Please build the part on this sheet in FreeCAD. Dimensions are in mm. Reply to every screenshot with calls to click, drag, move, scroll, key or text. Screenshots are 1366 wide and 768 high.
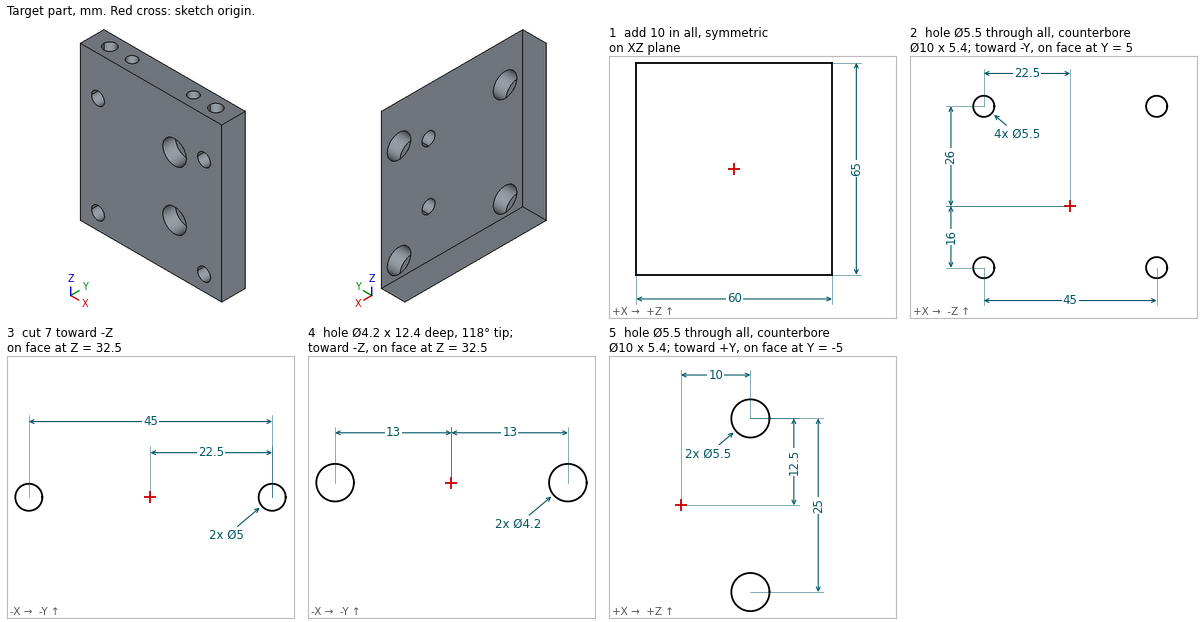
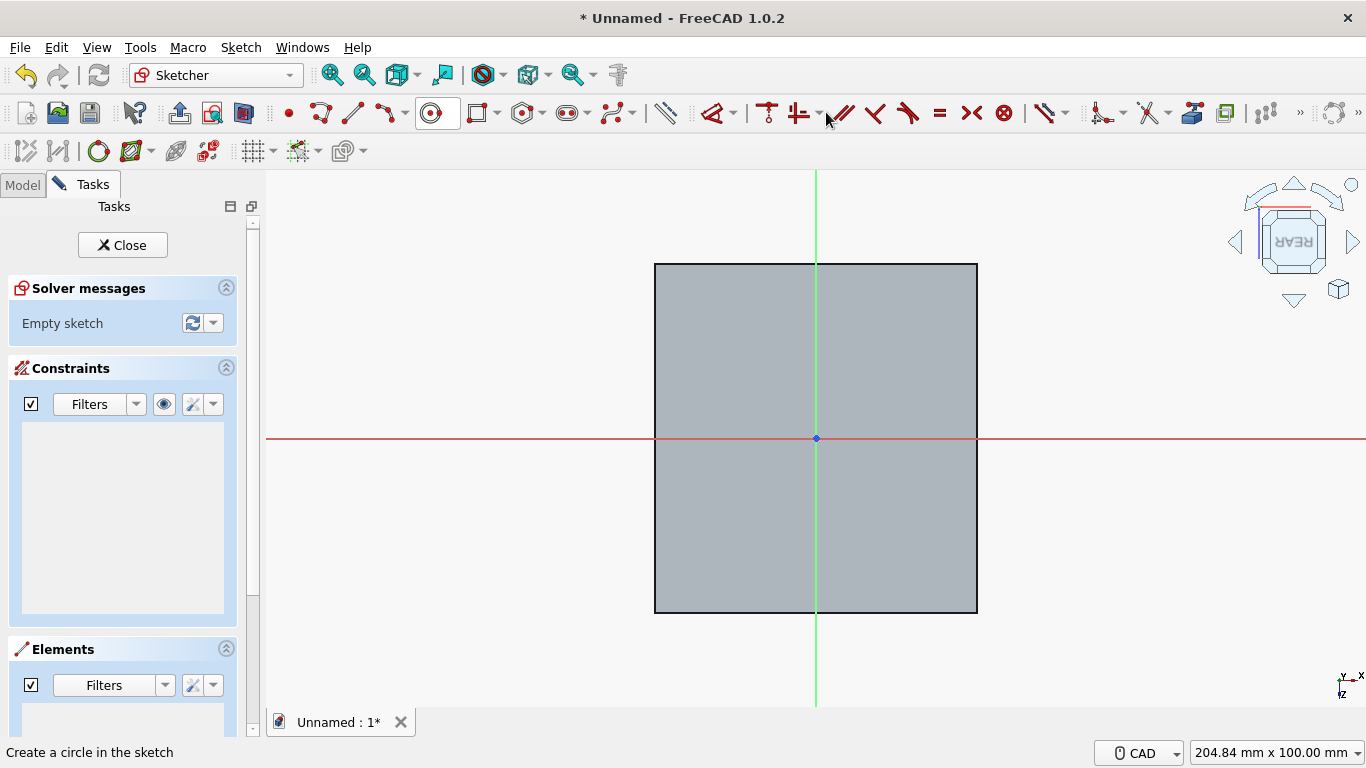
key(g)
key(c)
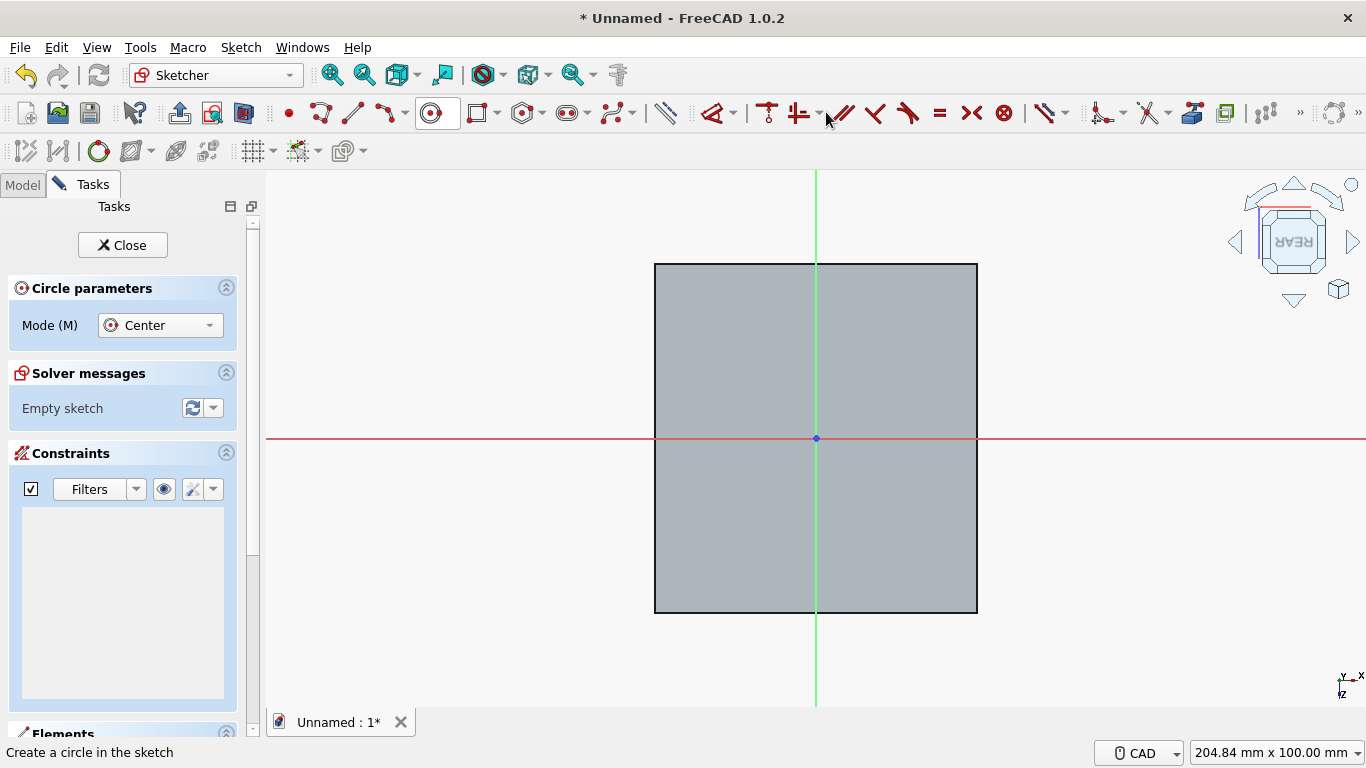
scroll(695, 299, up, 3)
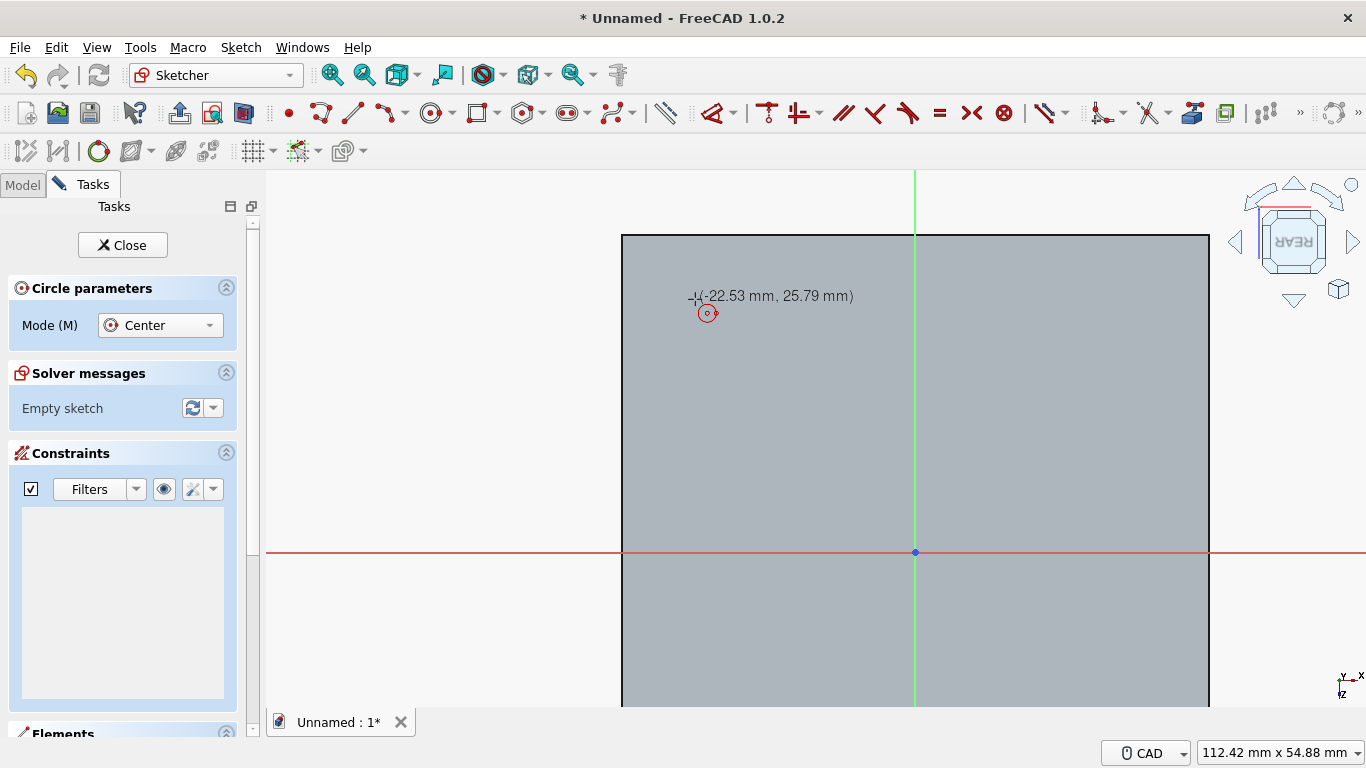
click(695, 299)
click(714, 280)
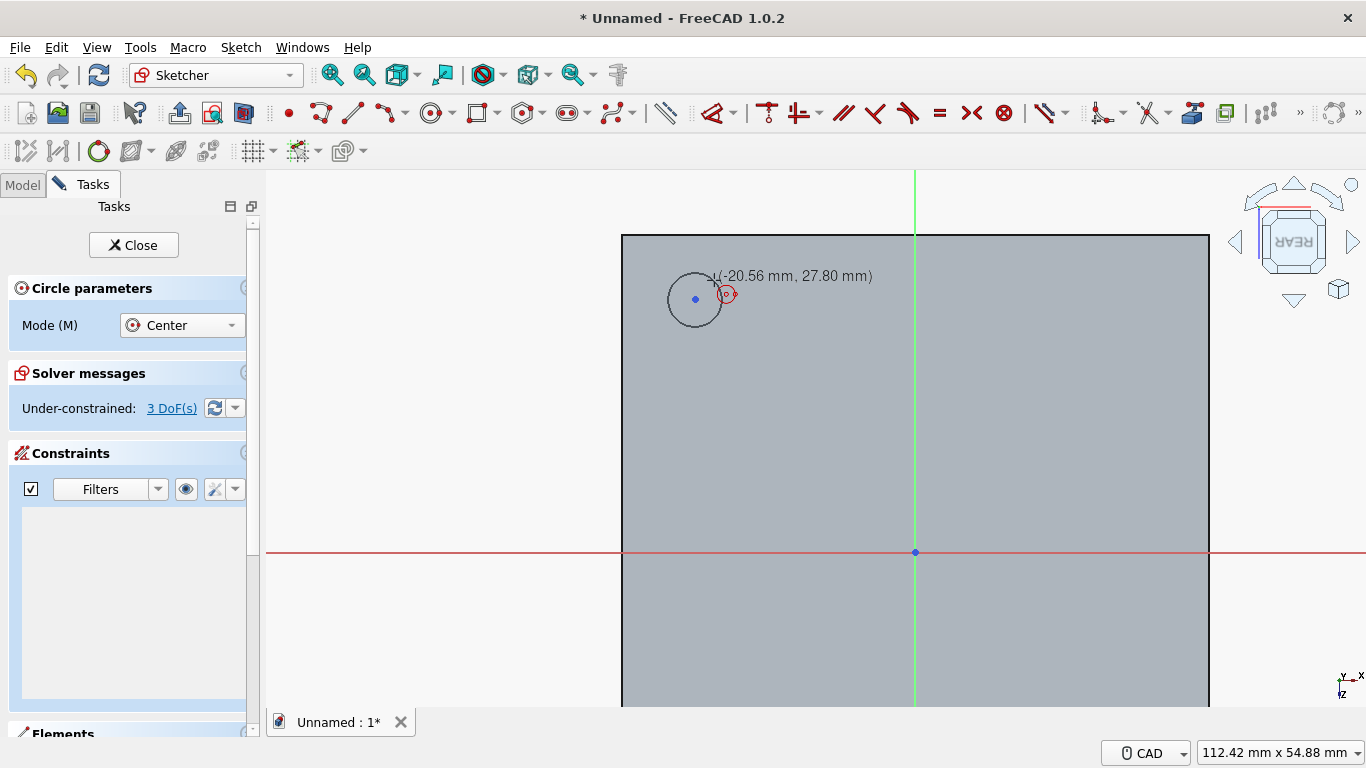
scroll(407, 305, down, 2)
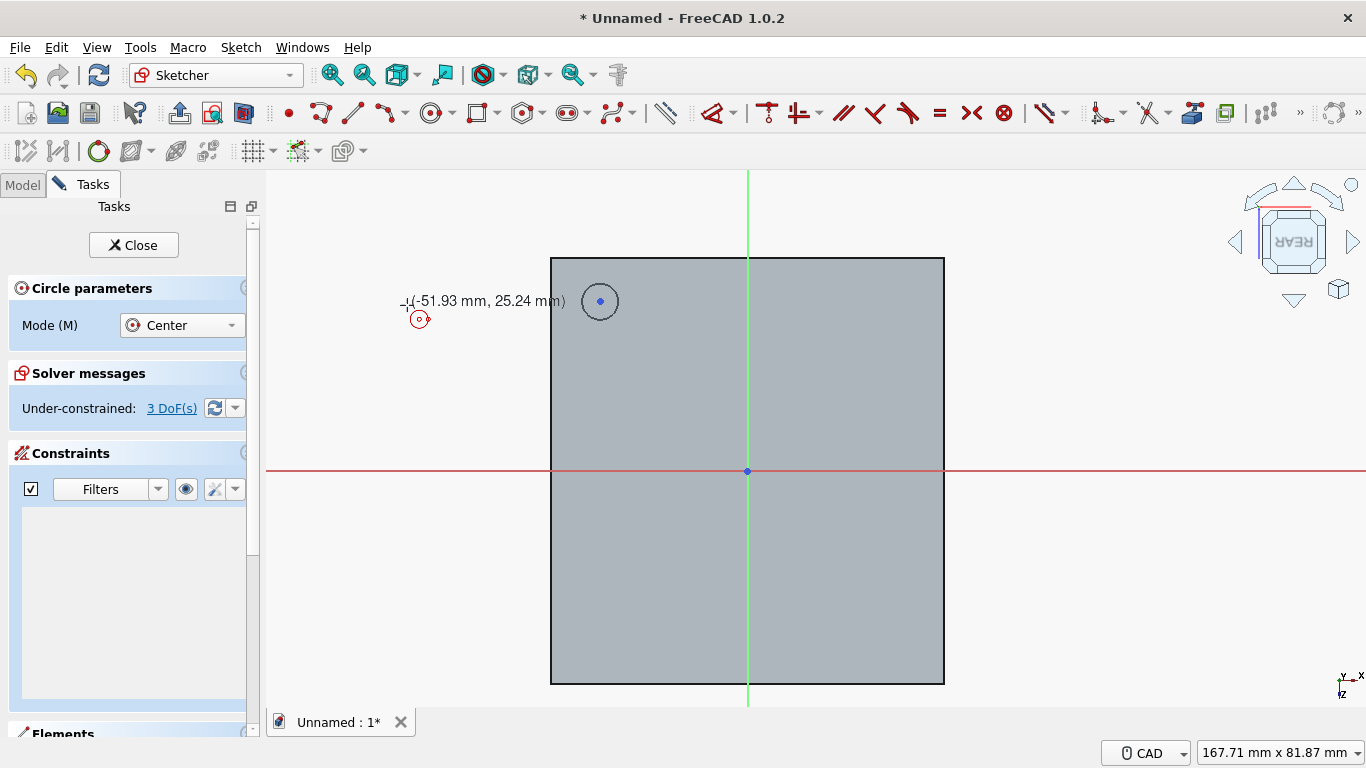
scroll(600, 576, up, 2)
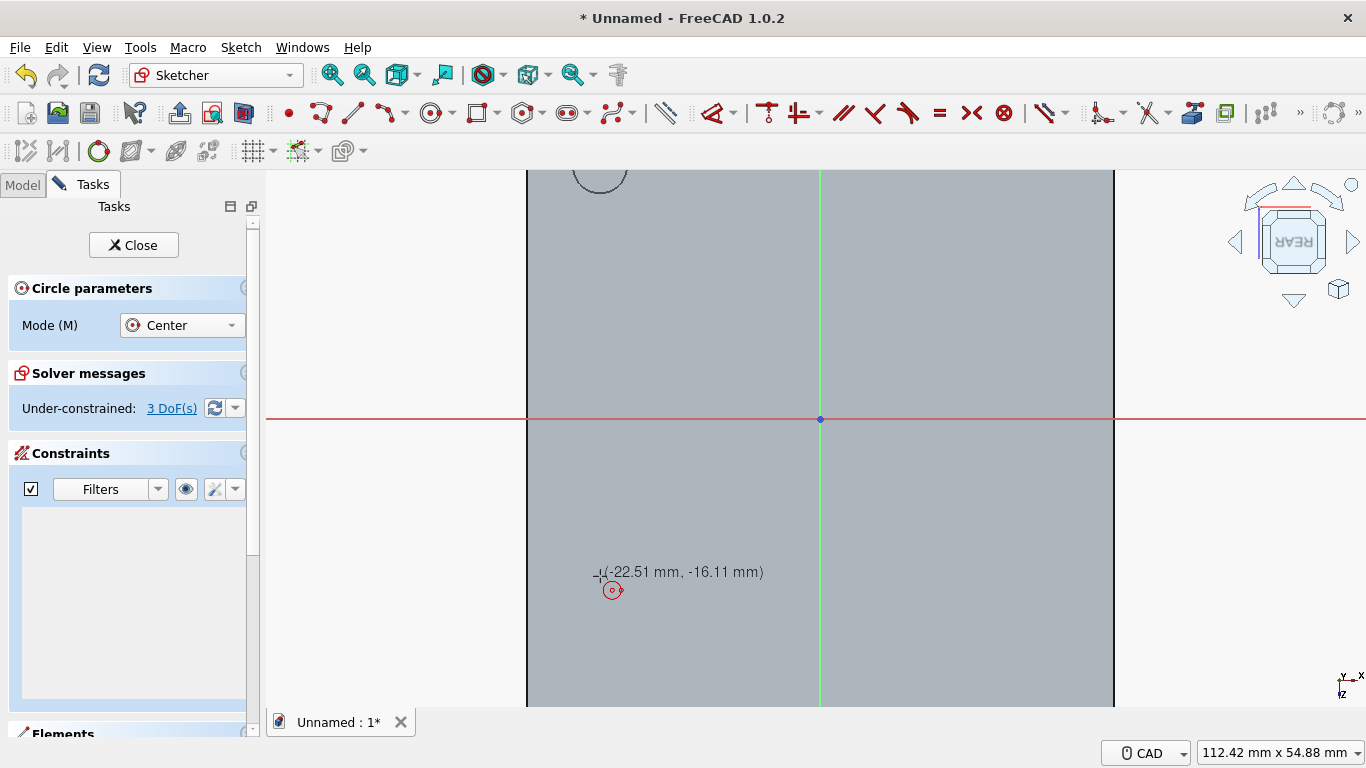
click(600, 576)
click(619, 557)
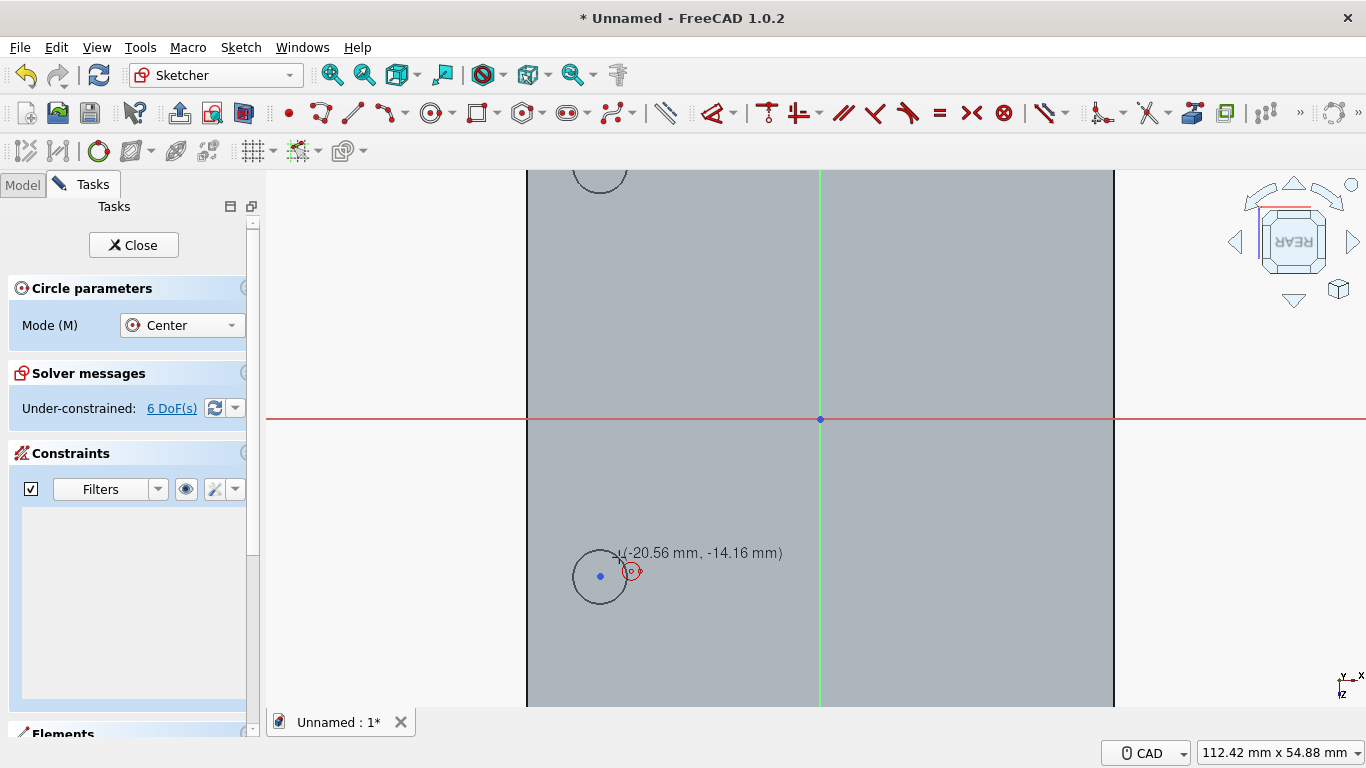
click(1040, 576)
click(1059, 557)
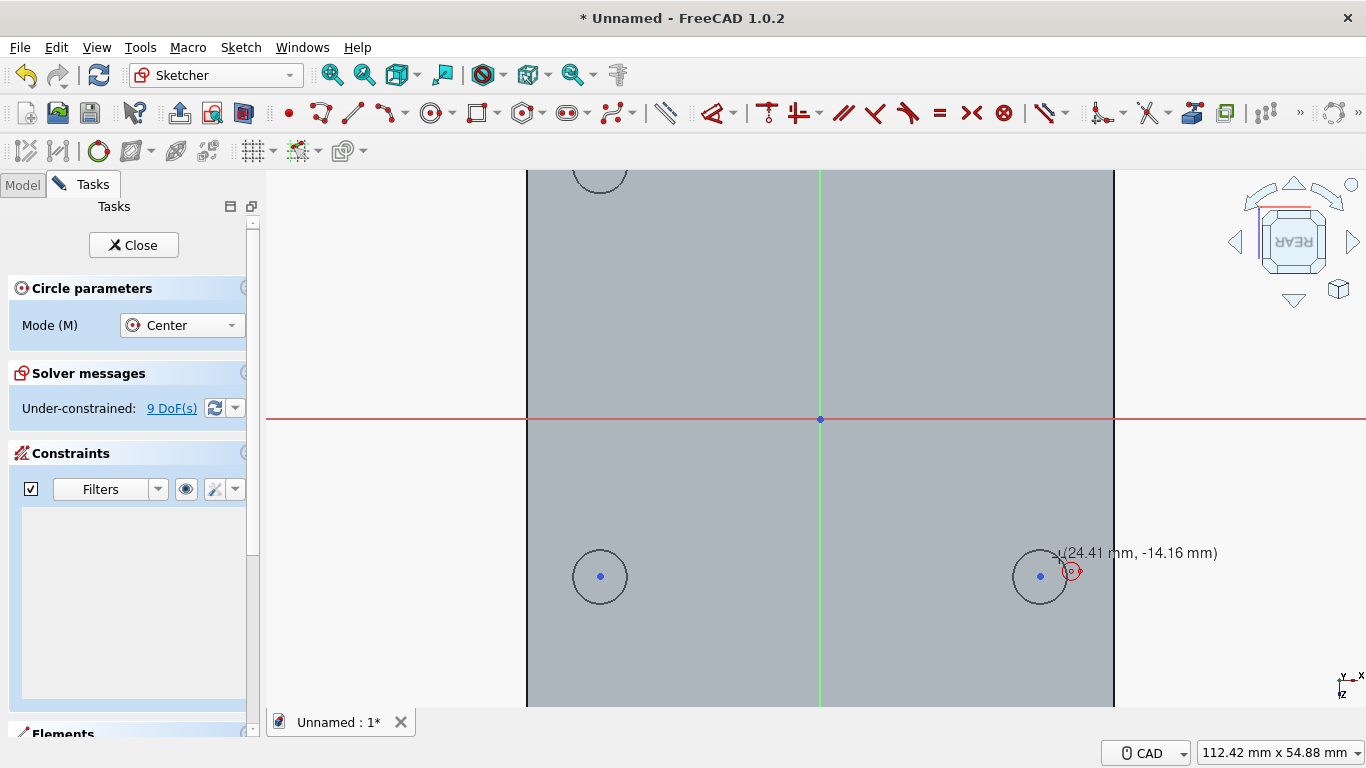
scroll(600, 577, down, 2)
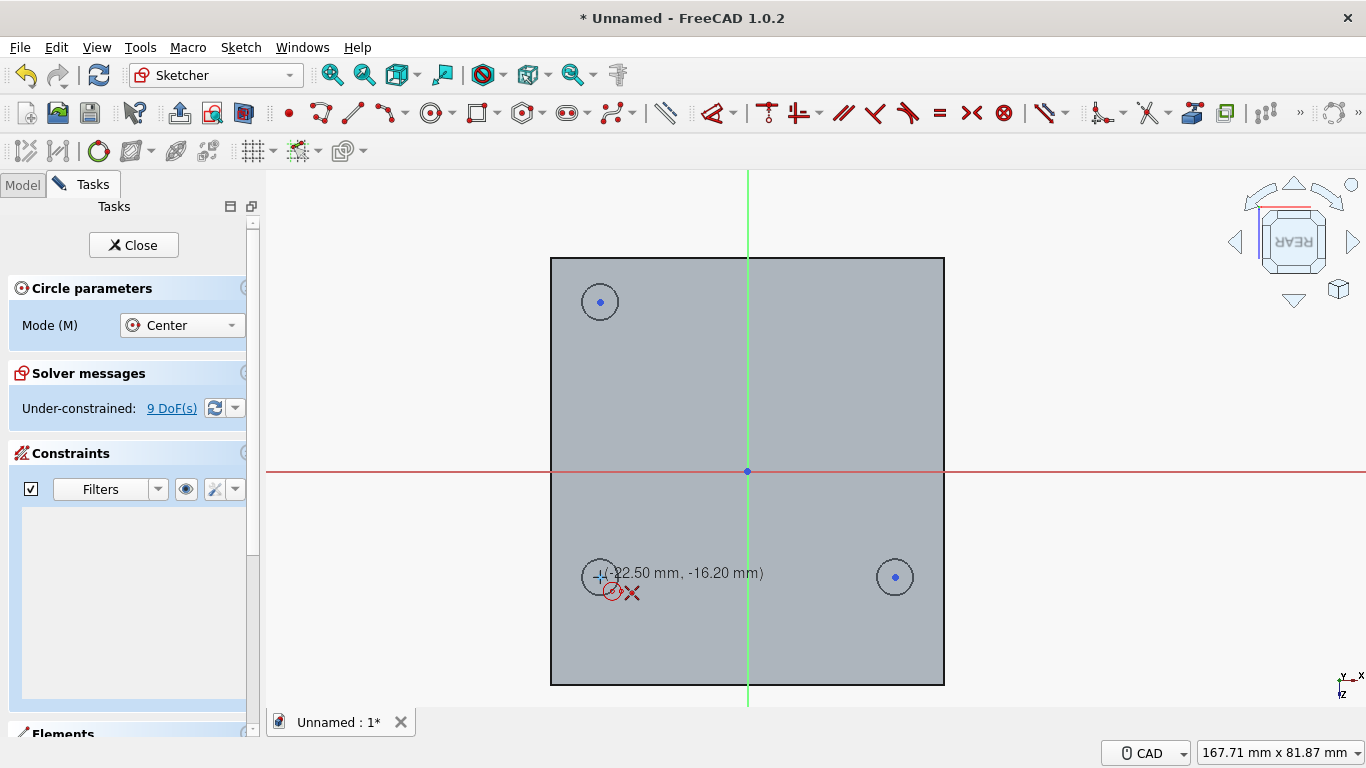
scroll(895, 301, up, 2)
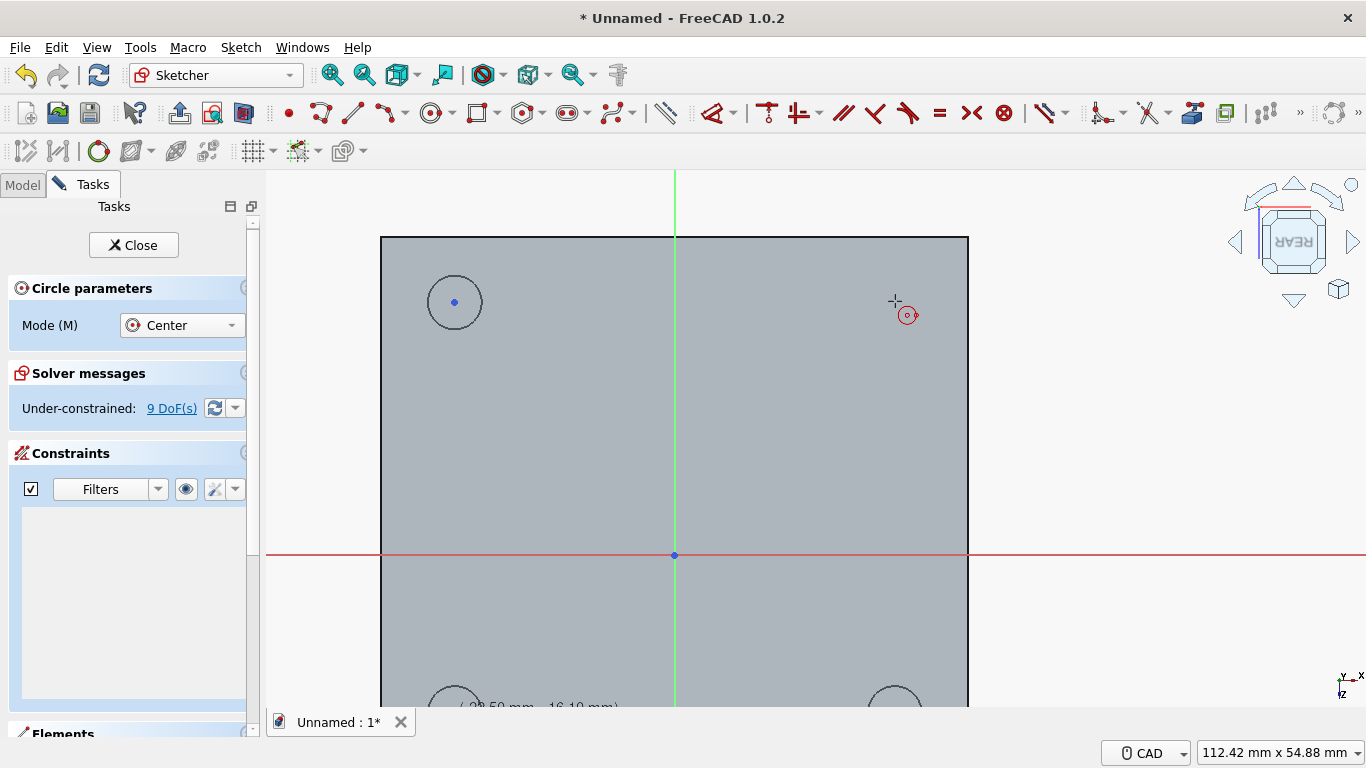
click(895, 301)
click(914, 282)
key(Escape)